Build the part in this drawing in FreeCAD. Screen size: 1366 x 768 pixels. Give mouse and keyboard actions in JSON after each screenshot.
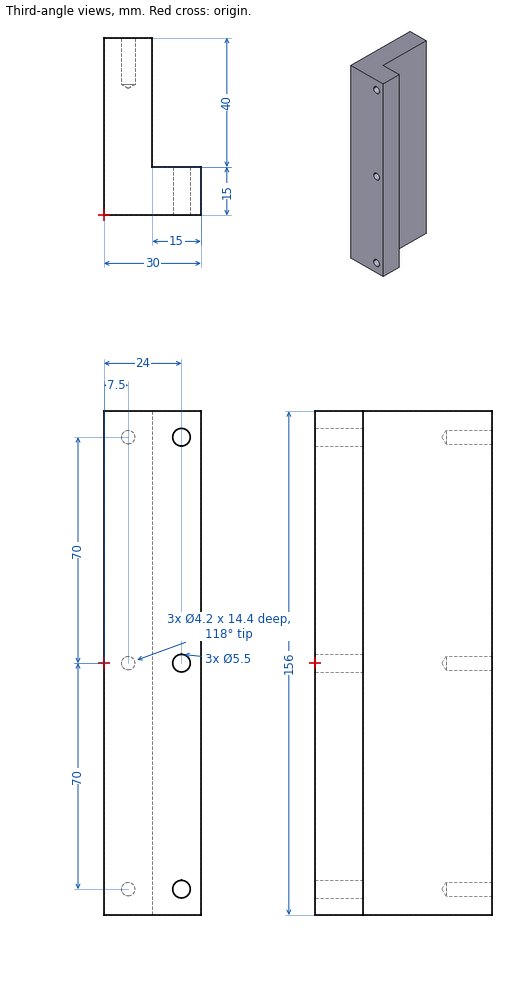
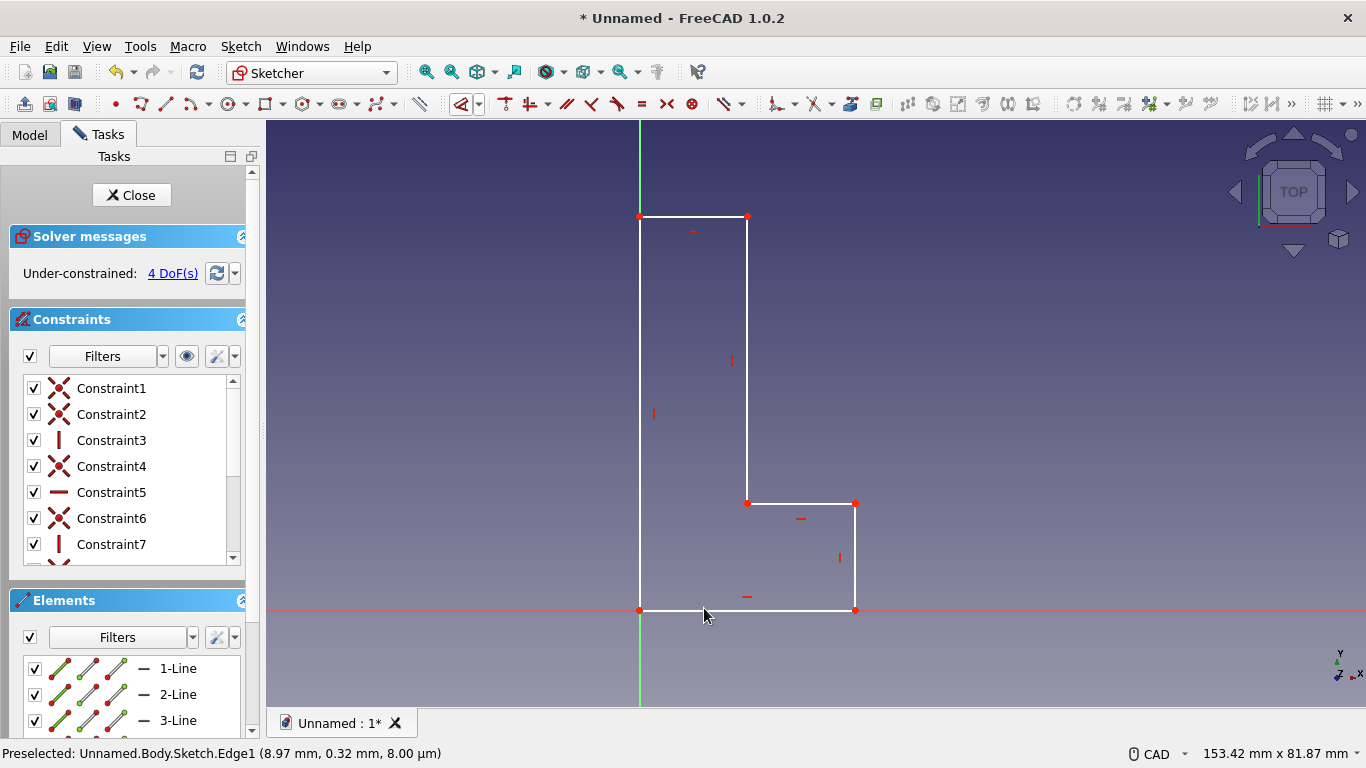
{"action": "left_click", "coordinate": [704, 611]}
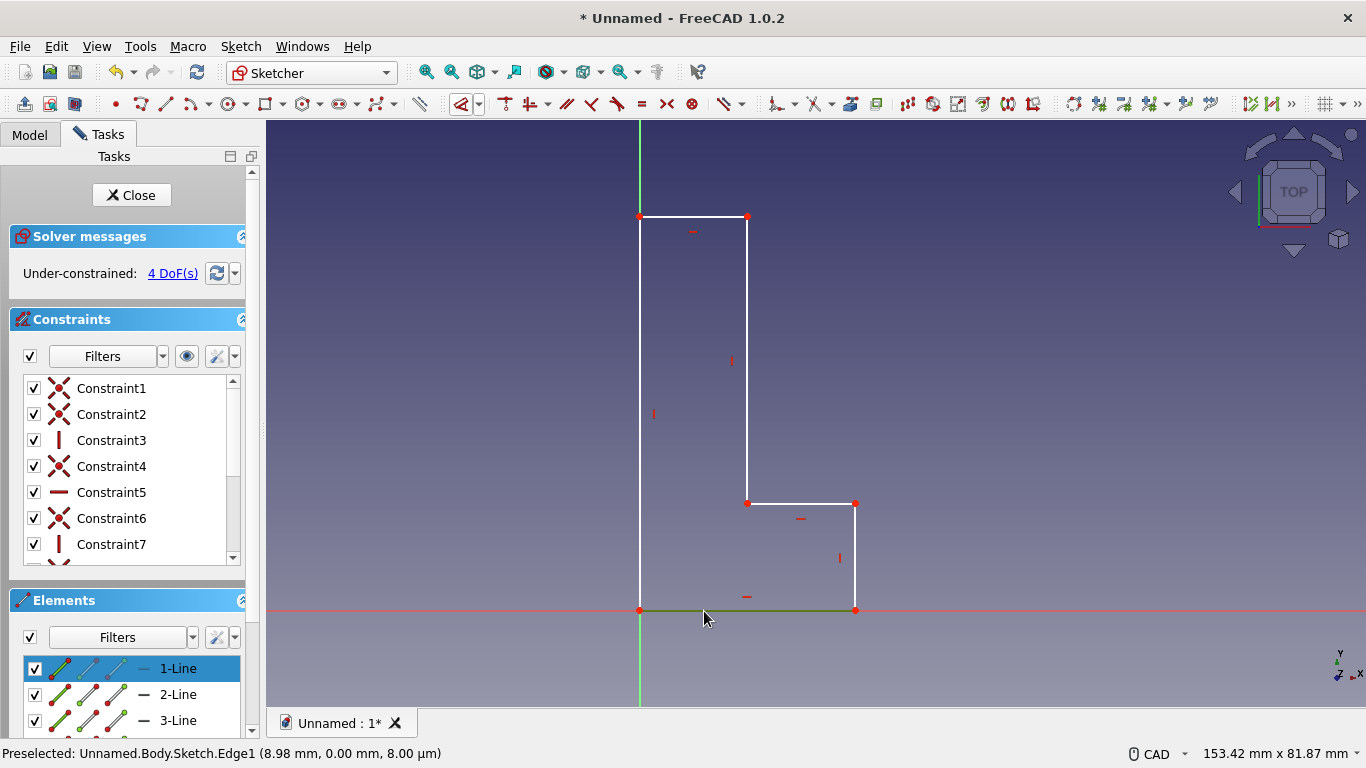
{"action": "key", "text": "l"}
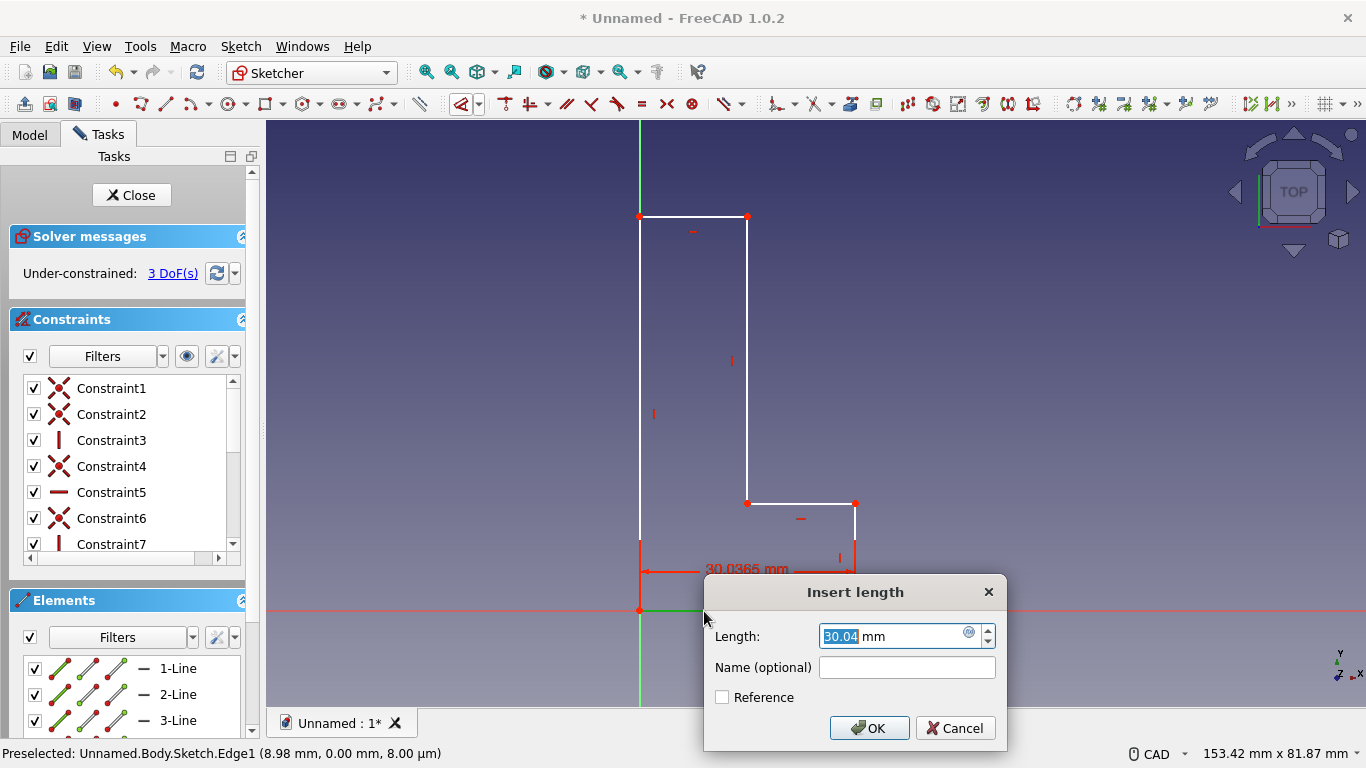
{"action": "type", "text": "30"}
{"action": "key", "text": "Return"}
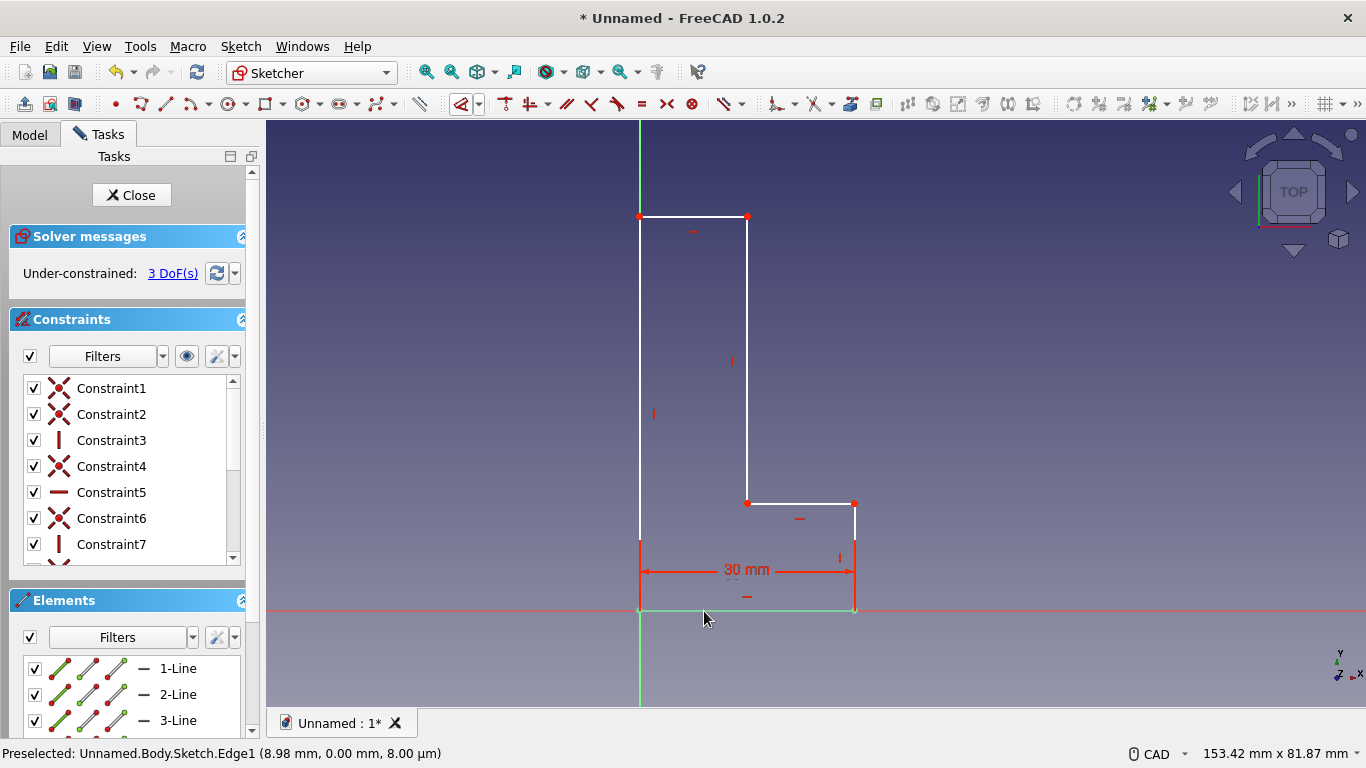
{"action": "left_click", "coordinate": [855, 579]}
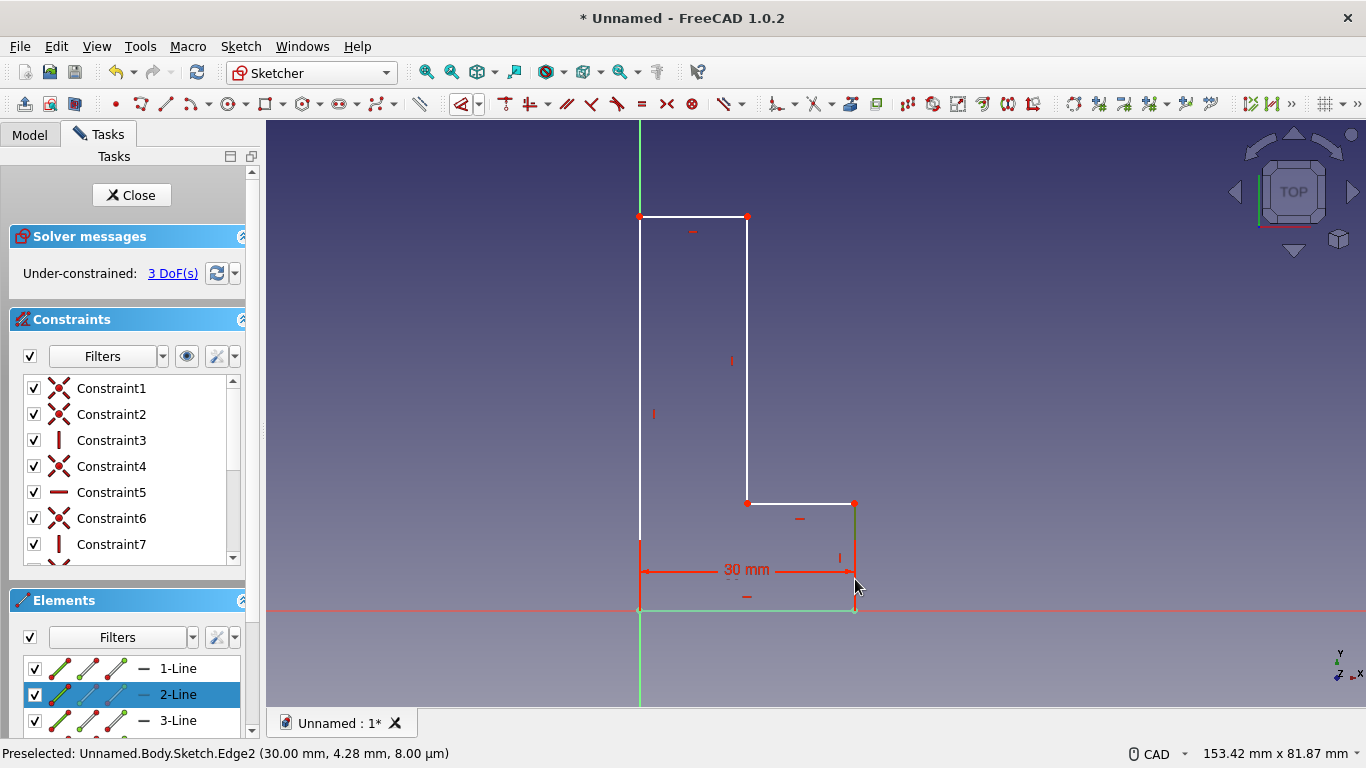
{"action": "key", "text": "i"}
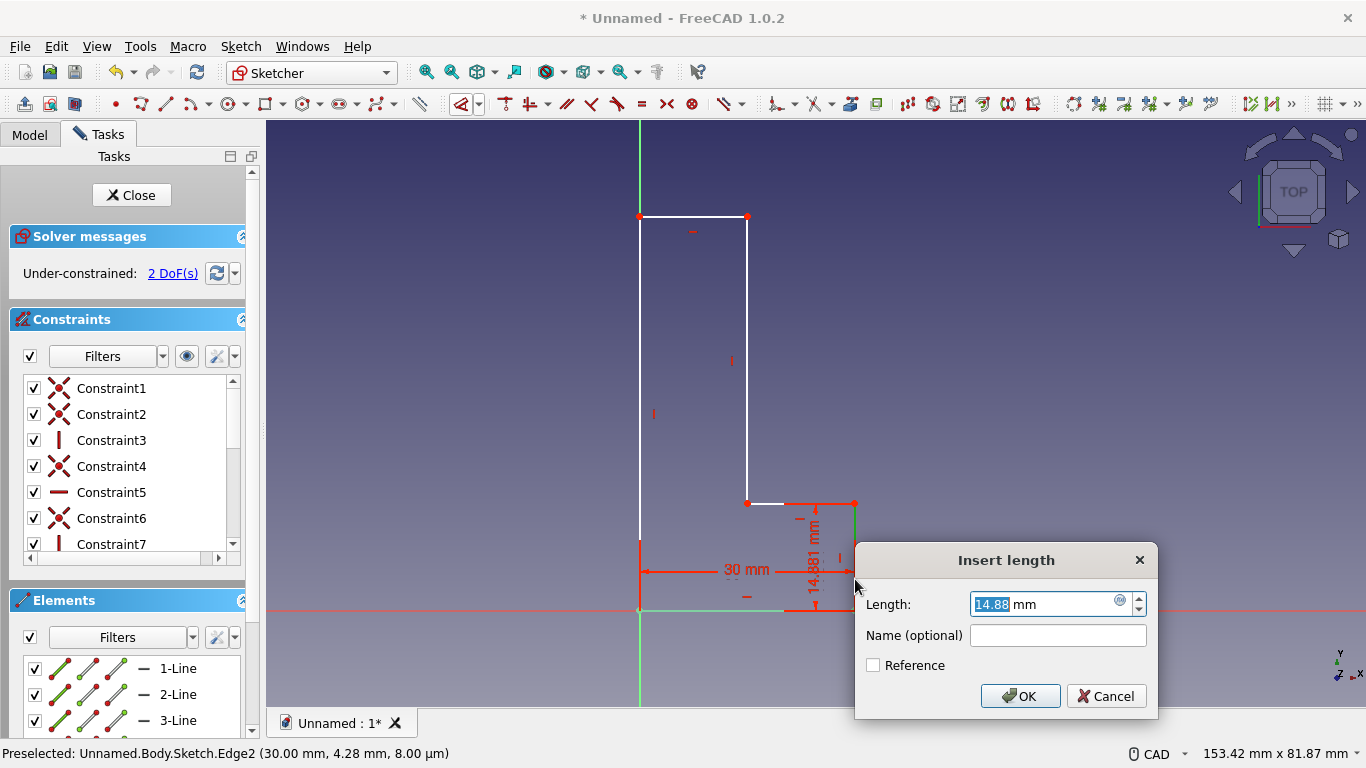
{"action": "type", "text": "15"}
{"action": "key", "text": "Return"}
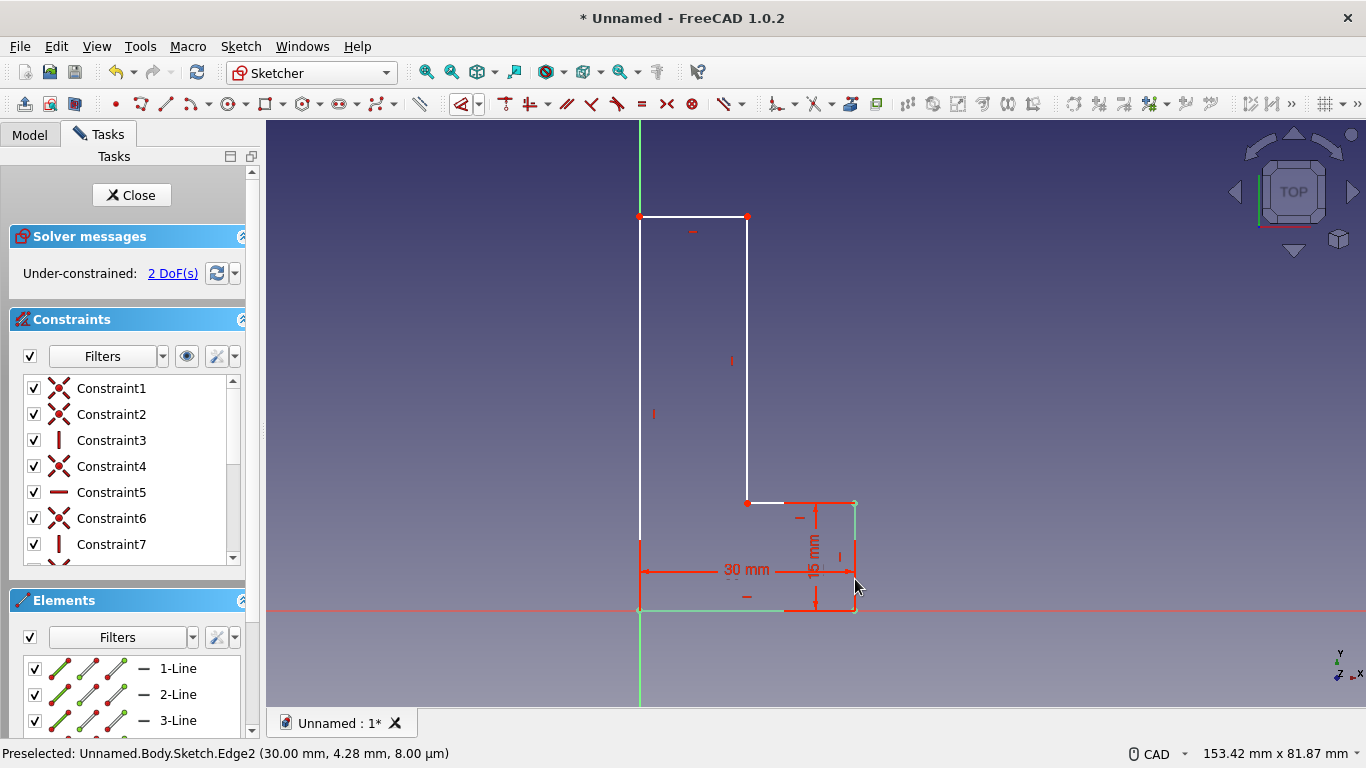
{"action": "left_click", "coordinate": [822, 503]}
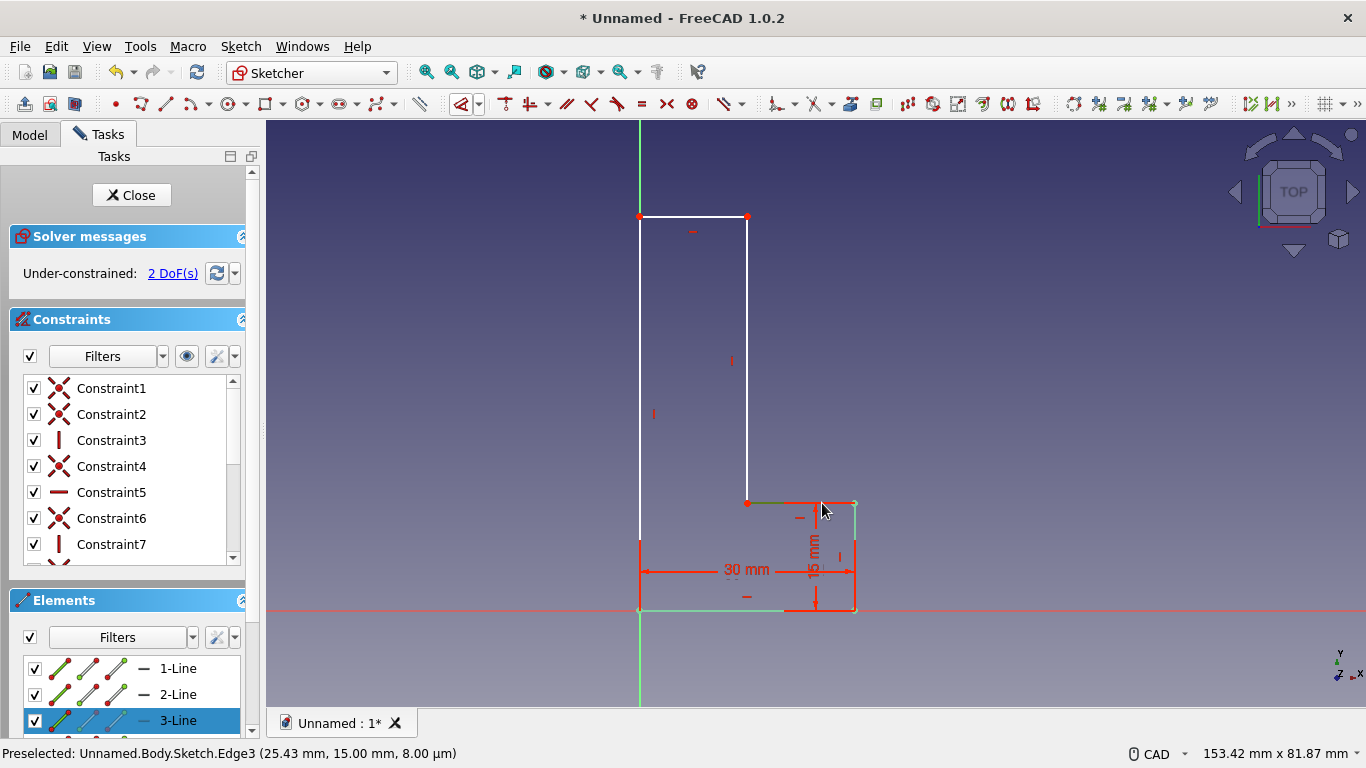
{"action": "key", "text": "l"}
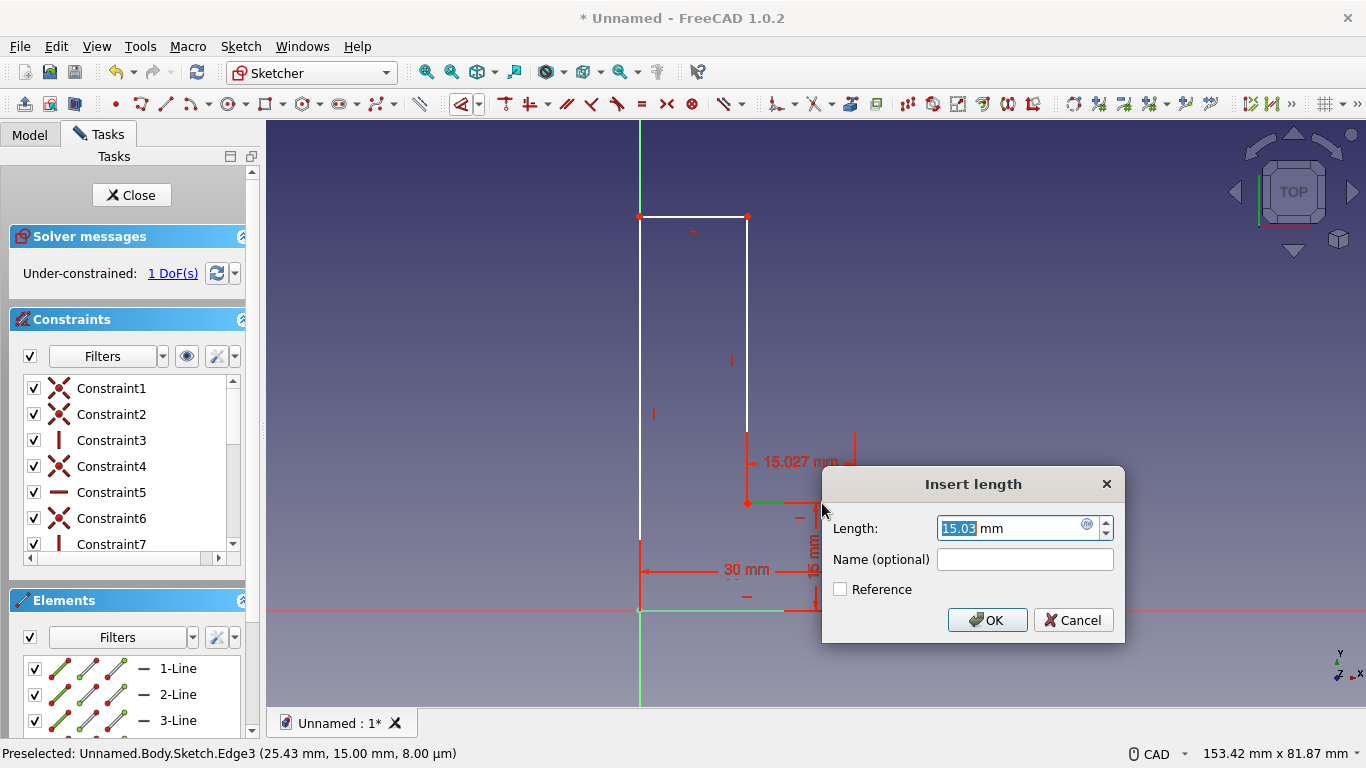
{"action": "type", "text": "15"}
{"action": "key", "text": "Return"}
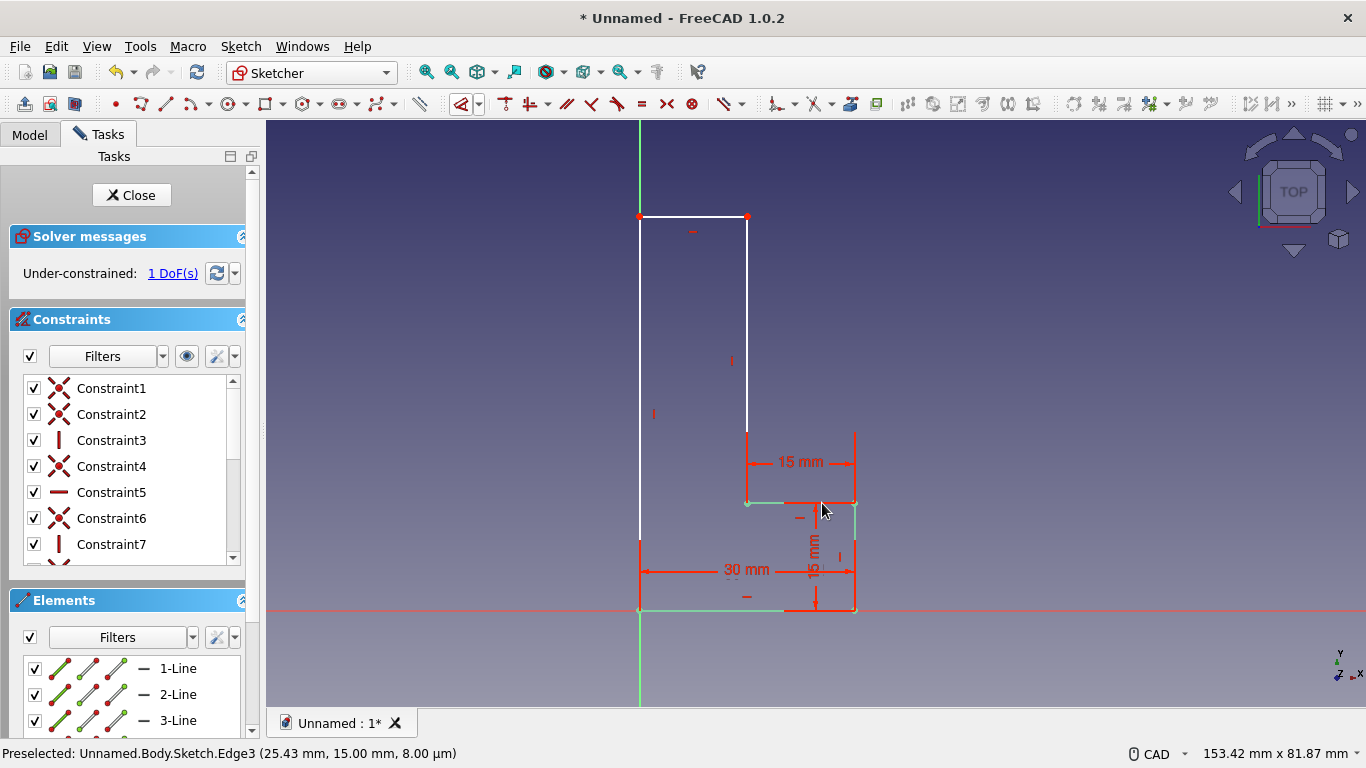
{"action": "left_click", "coordinate": [747, 417]}